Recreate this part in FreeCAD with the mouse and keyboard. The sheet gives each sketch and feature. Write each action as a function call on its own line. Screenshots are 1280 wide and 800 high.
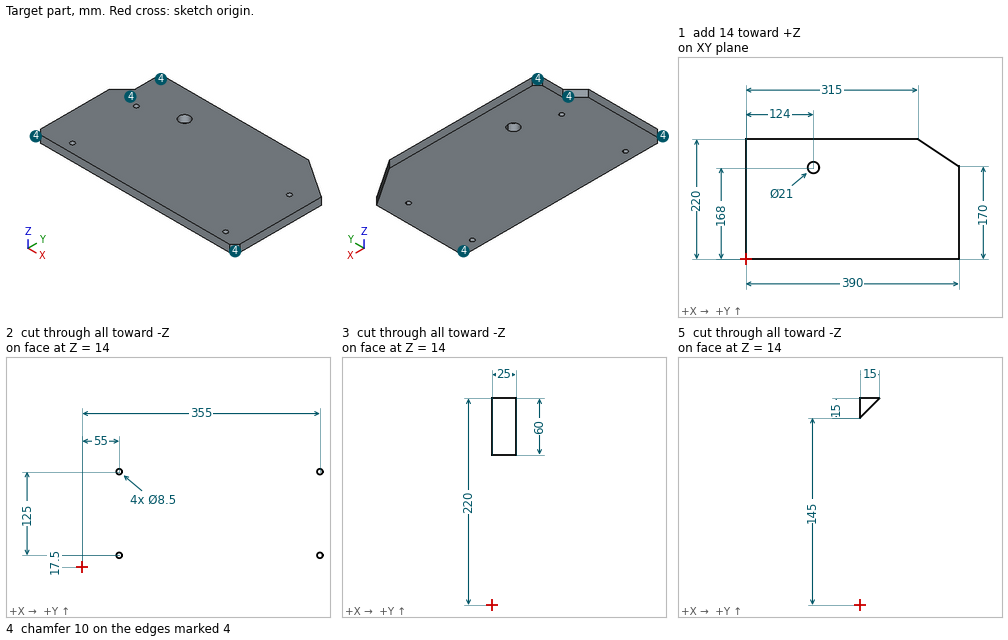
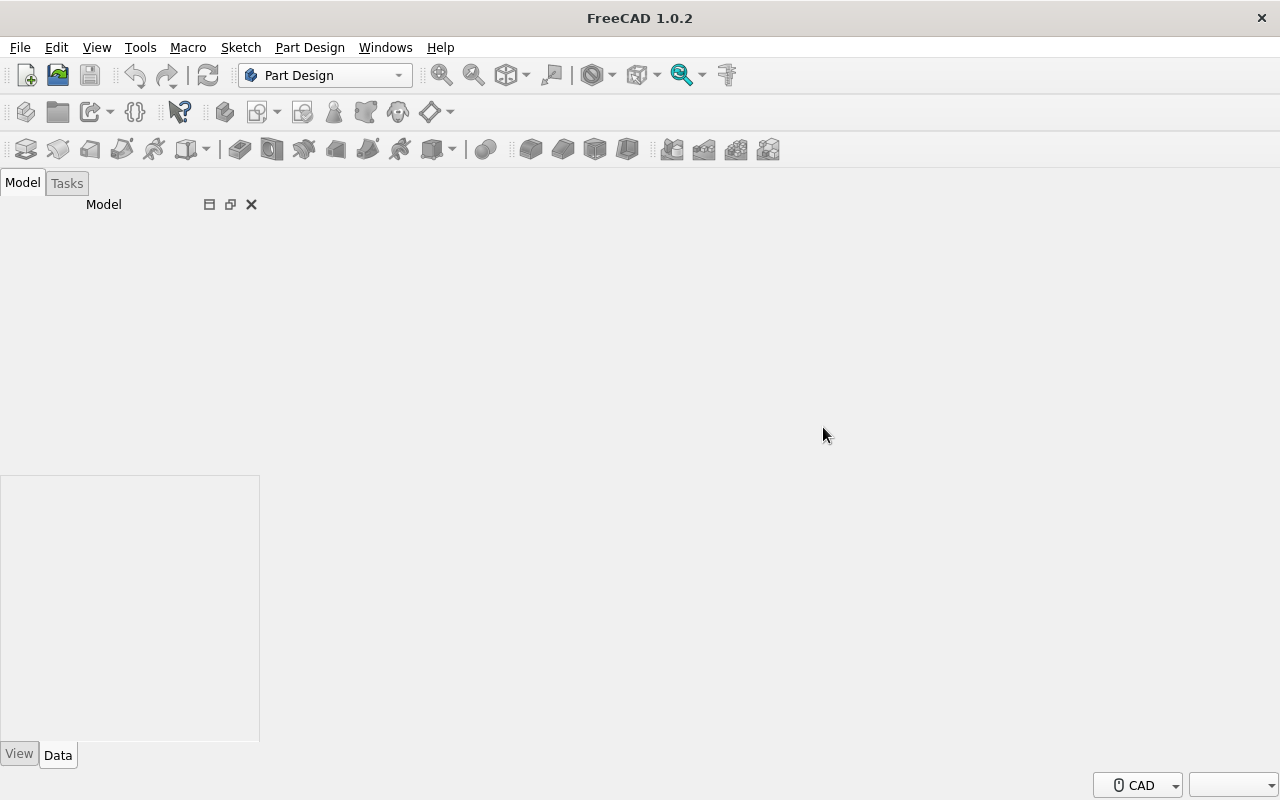
click(26, 76)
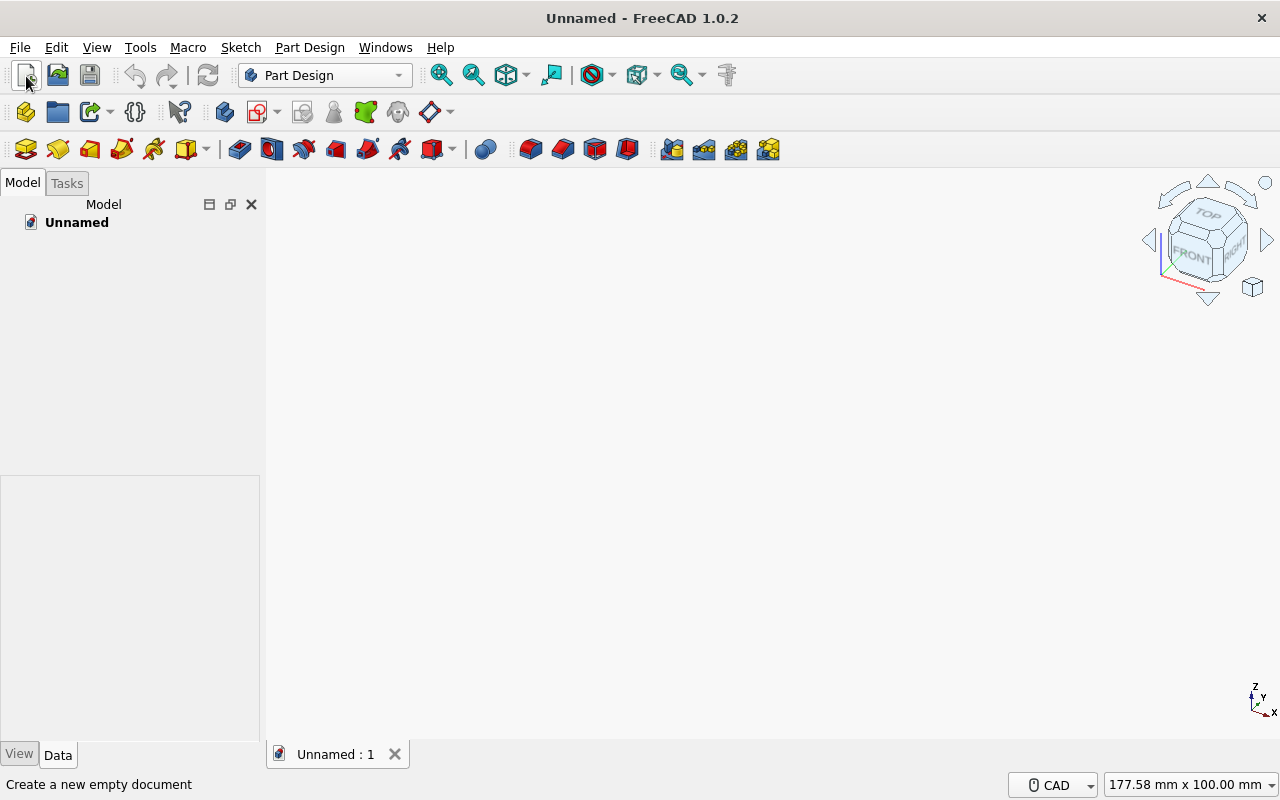
click(258, 112)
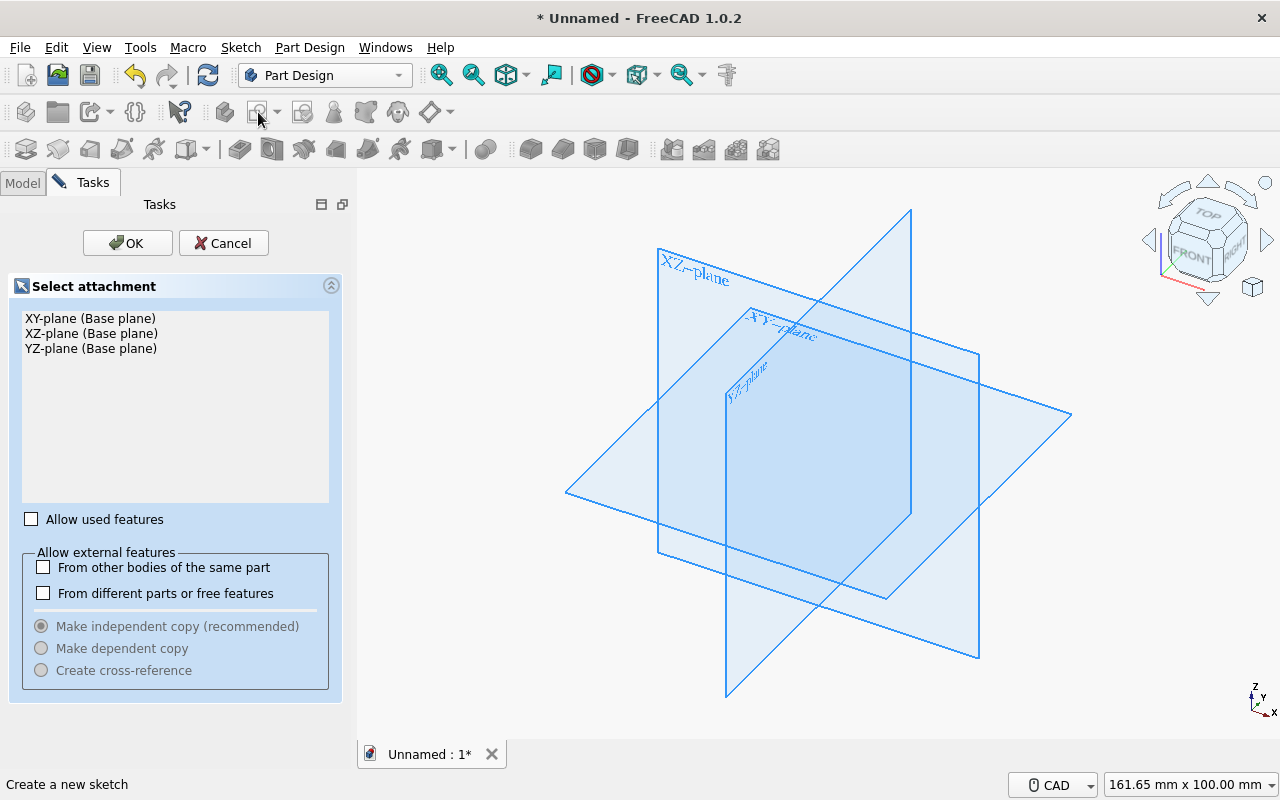
click(82, 318)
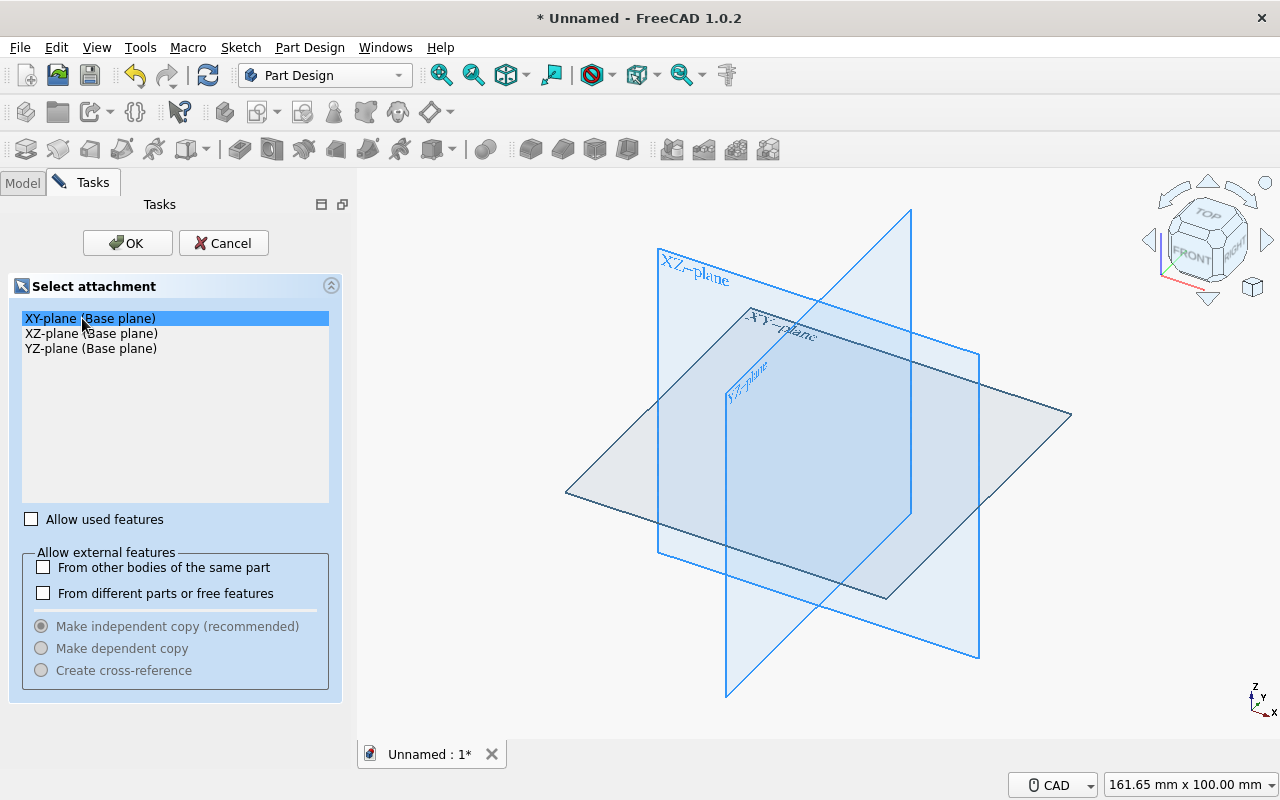
click(128, 243)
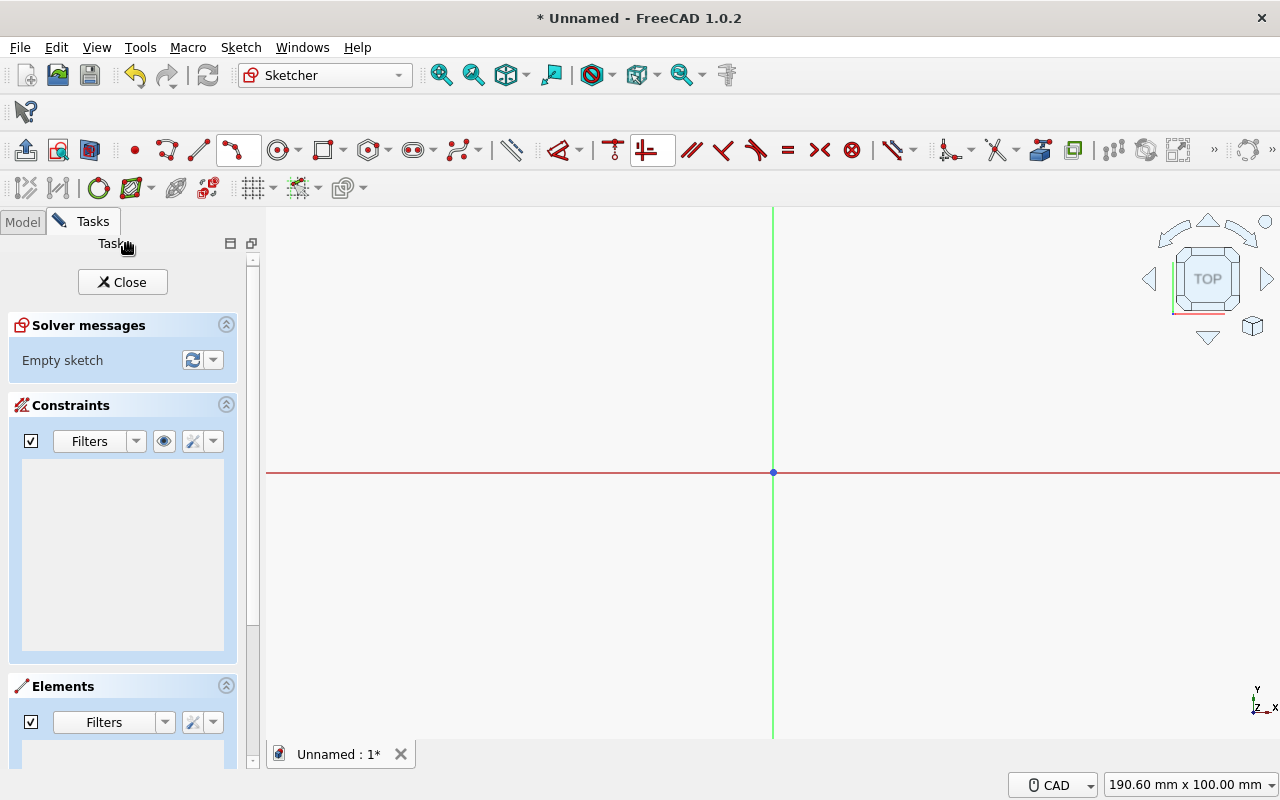
scroll(294, 711, down, 6)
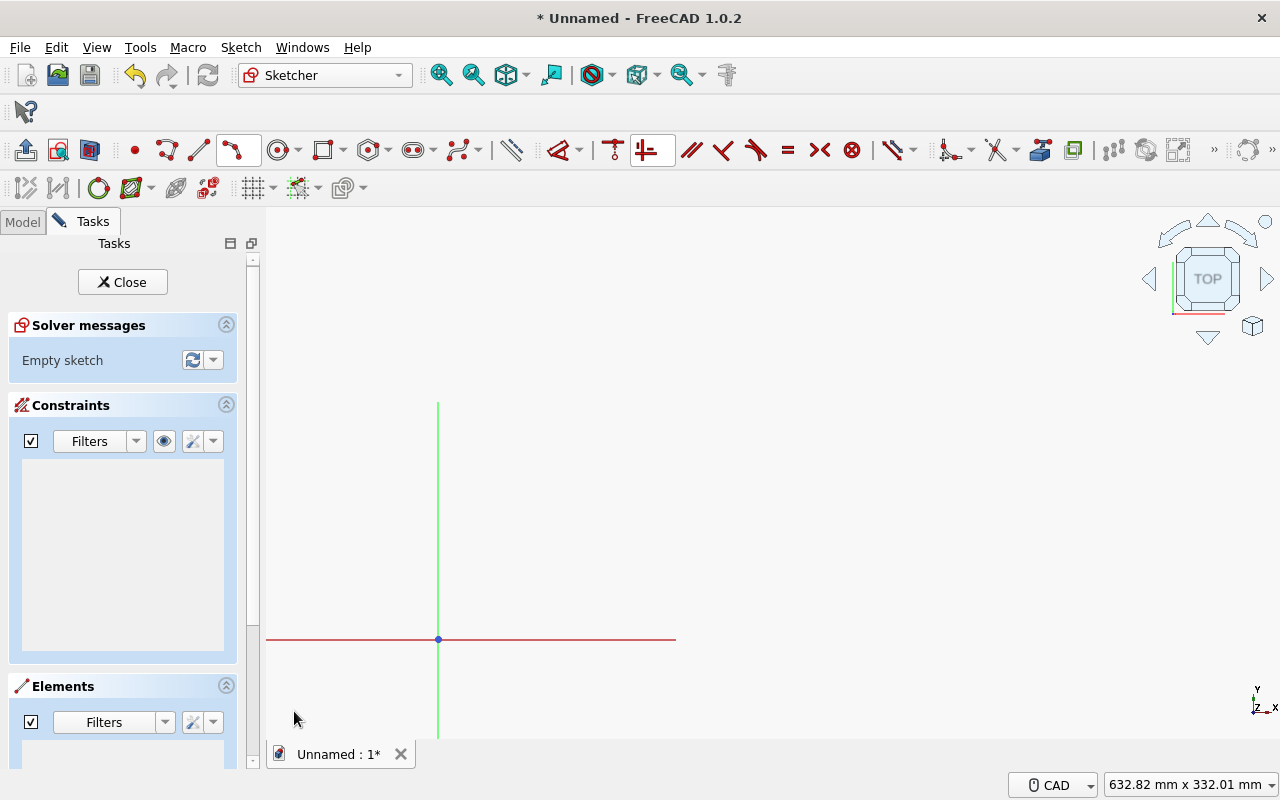
click(168, 150)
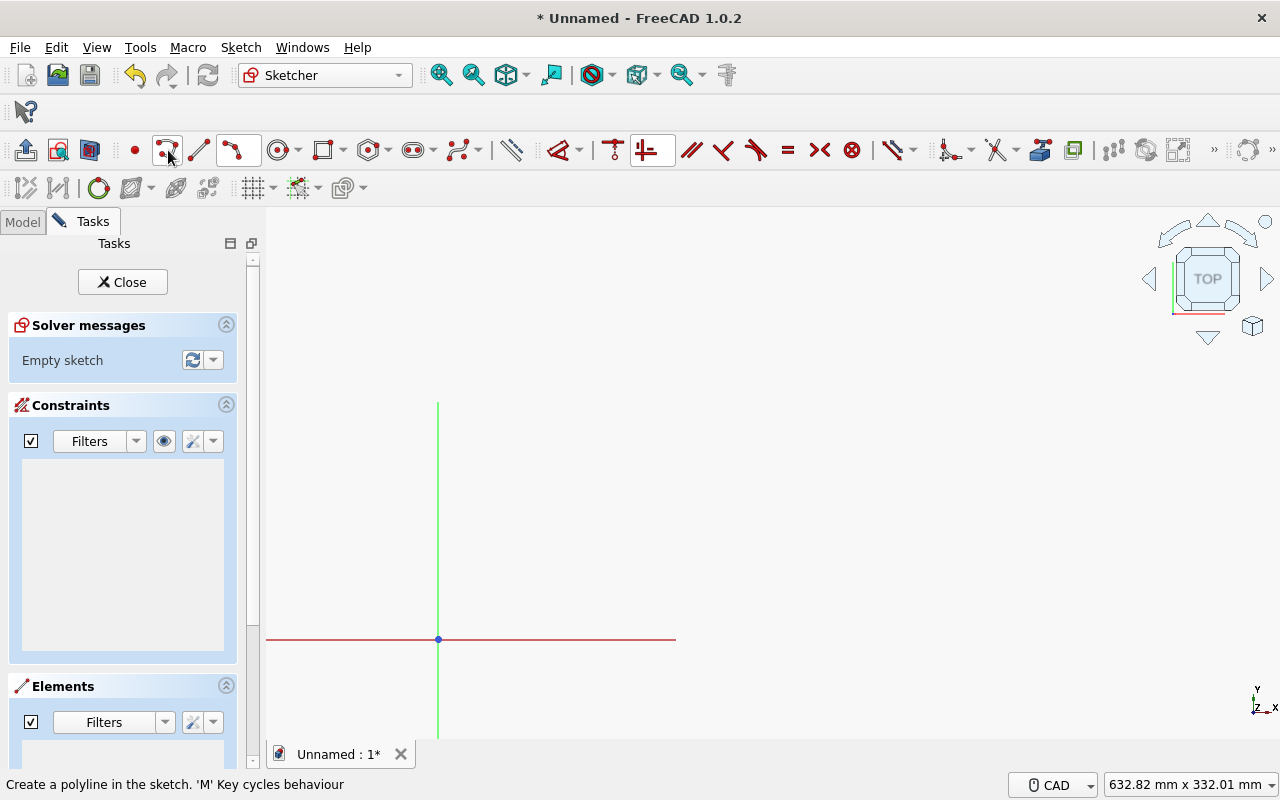
click(438, 640)
click(1063, 631)
click(1063, 368)
click(943, 287)
click(447, 287)
click(438, 640)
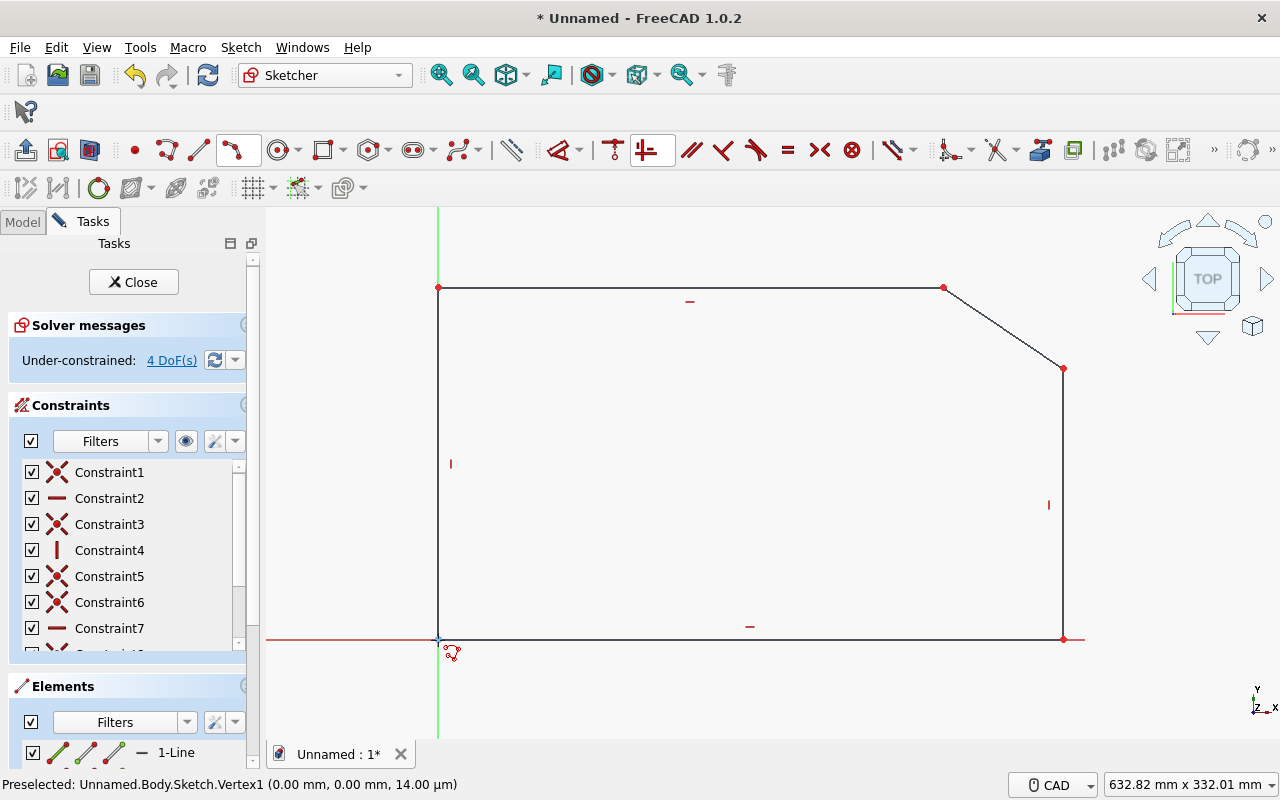
key(g)
key(c)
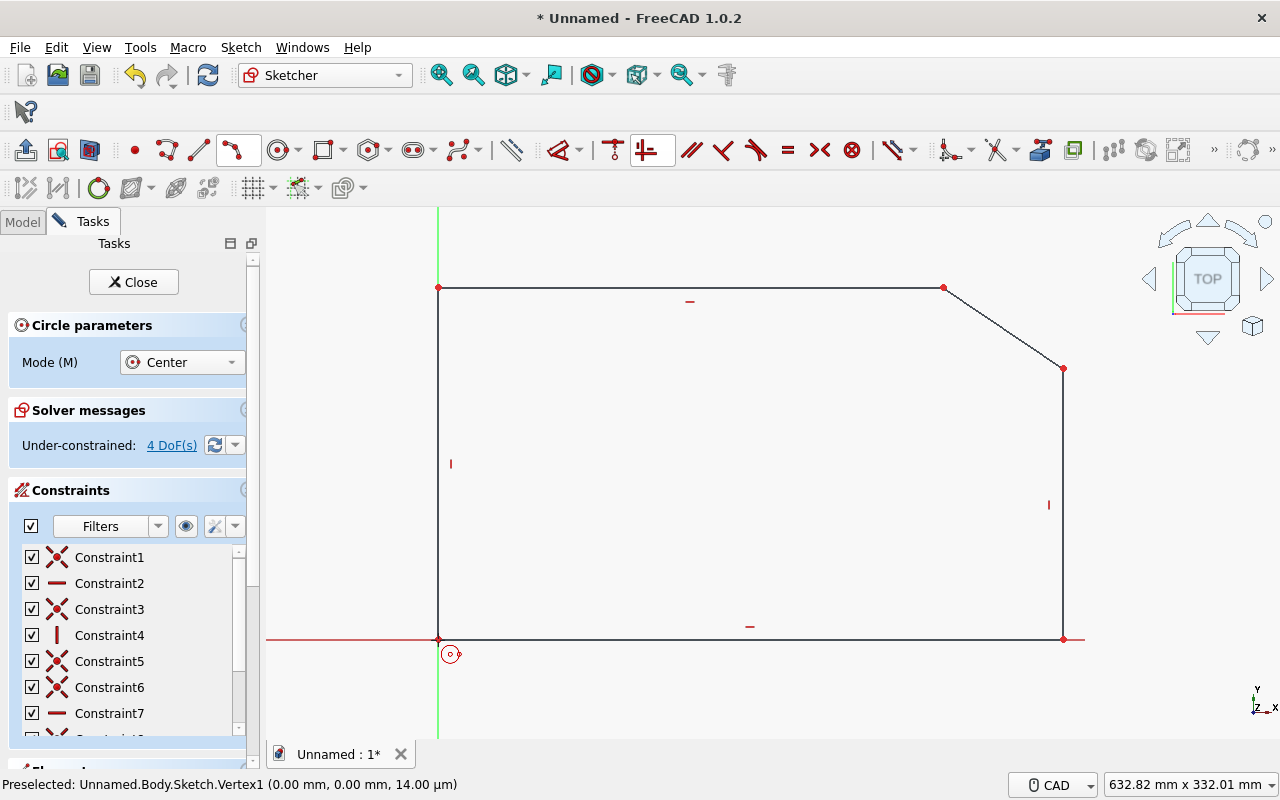
scroll(637, 371, up, 2)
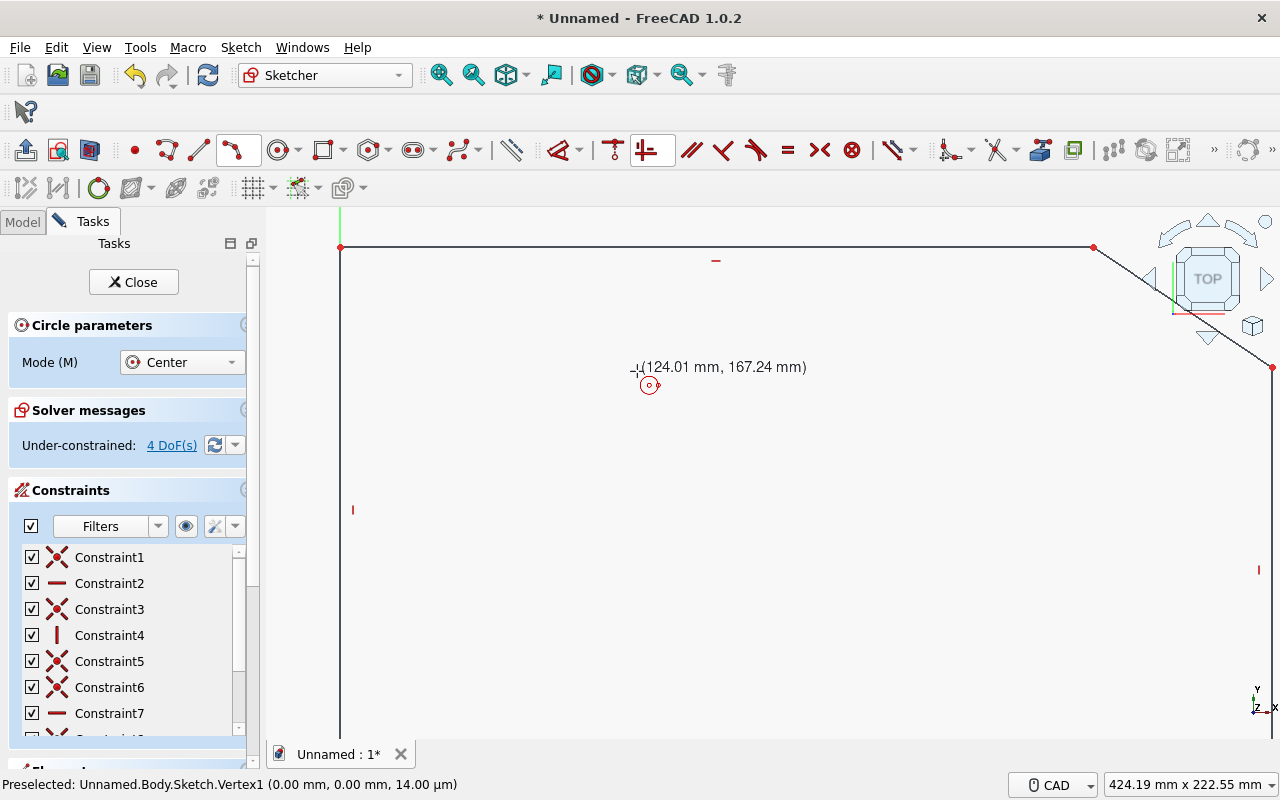
click(637, 371)
move(655, 353)